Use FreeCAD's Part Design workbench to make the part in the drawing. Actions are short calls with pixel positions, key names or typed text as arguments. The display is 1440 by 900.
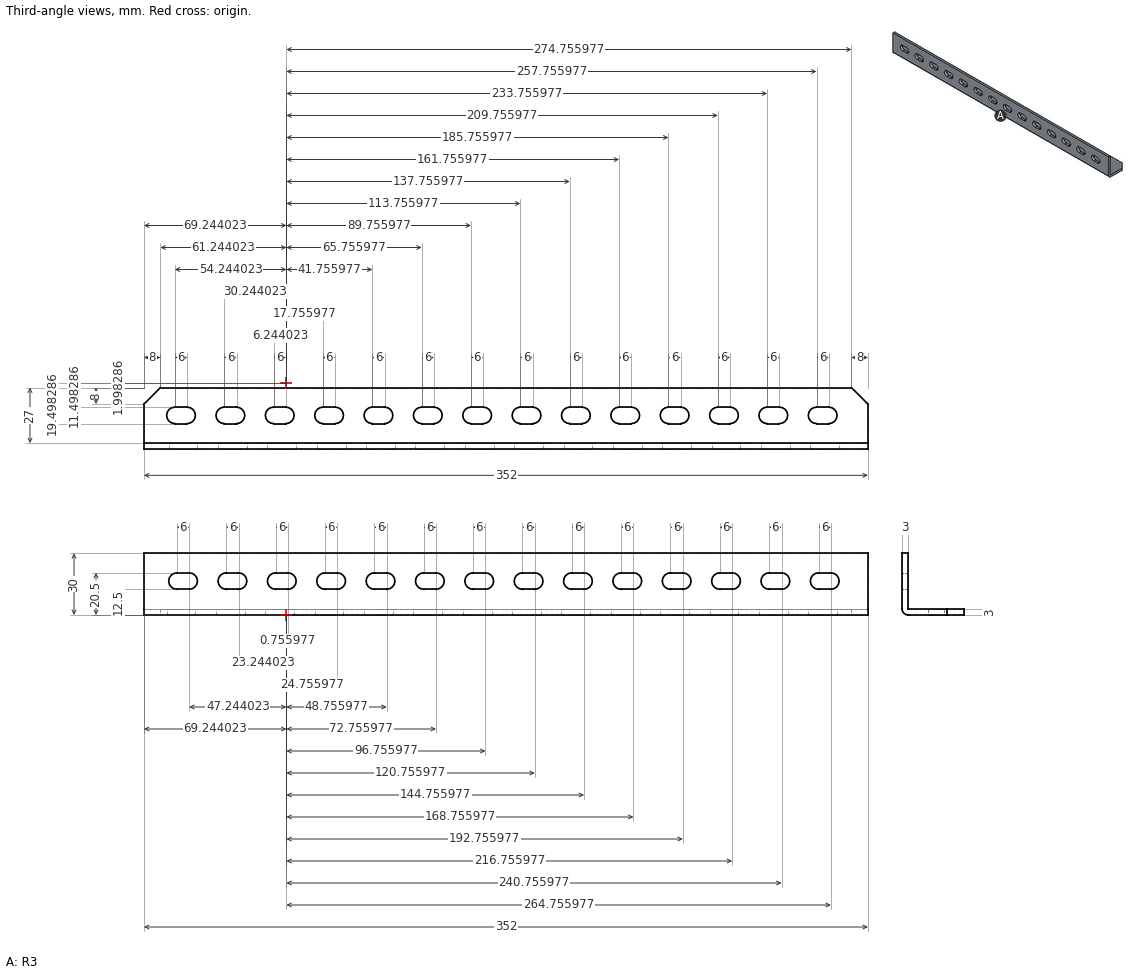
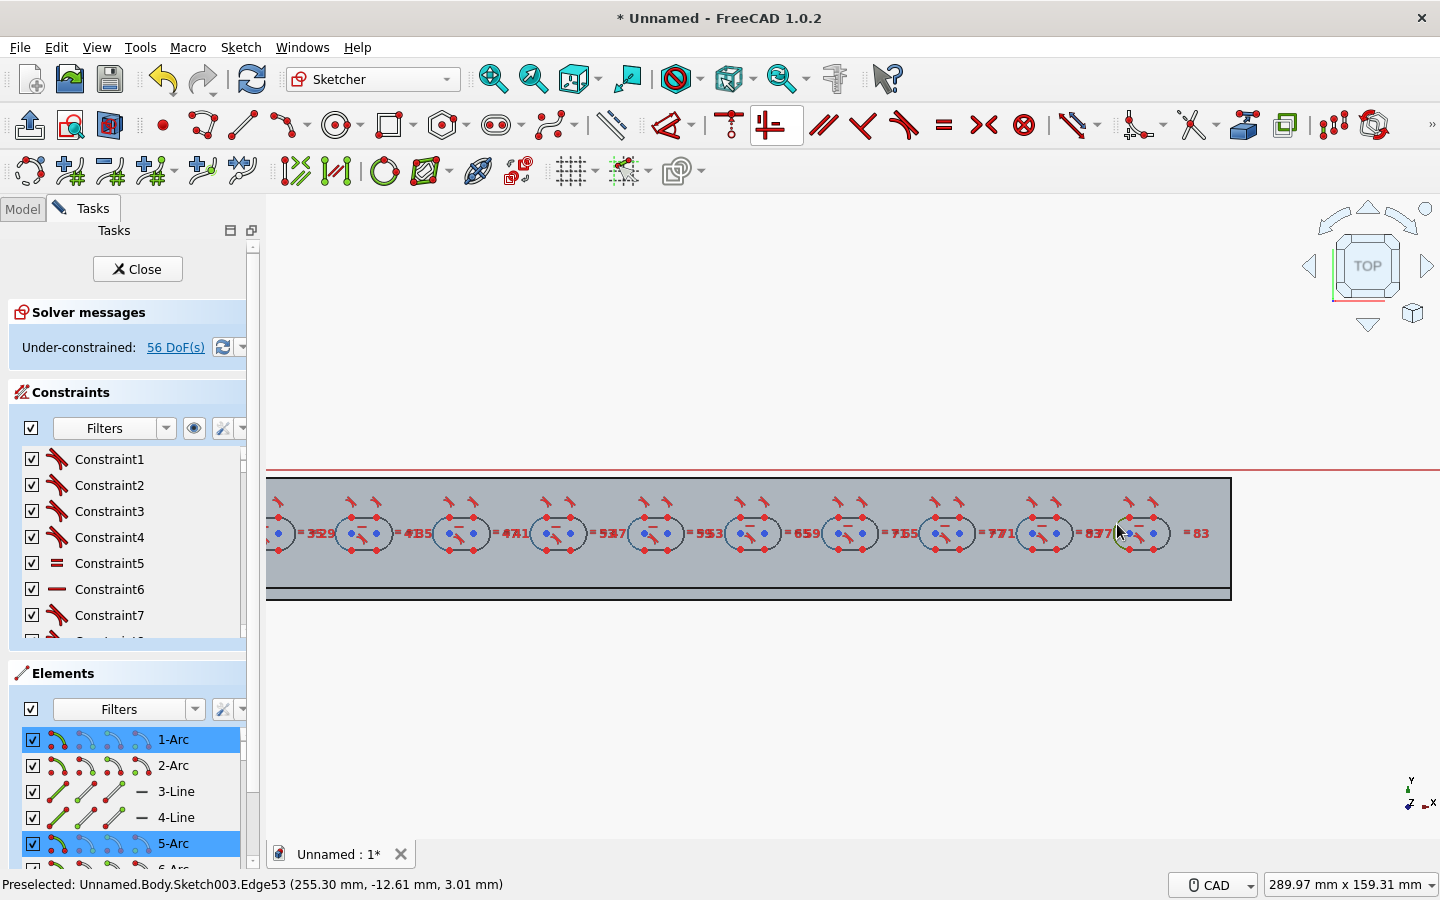
click(944, 126)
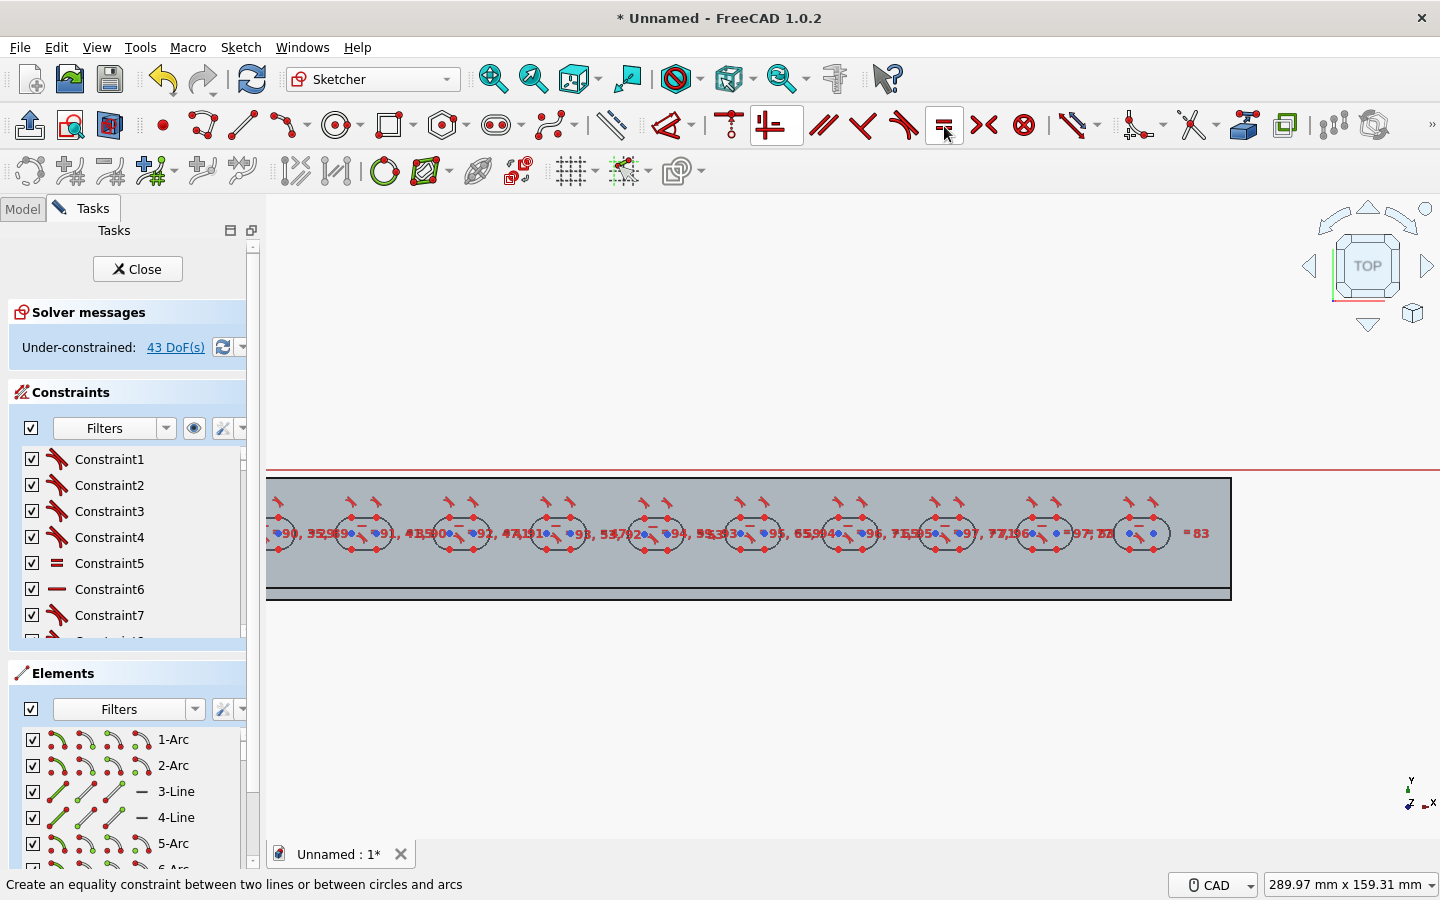
click(666, 126)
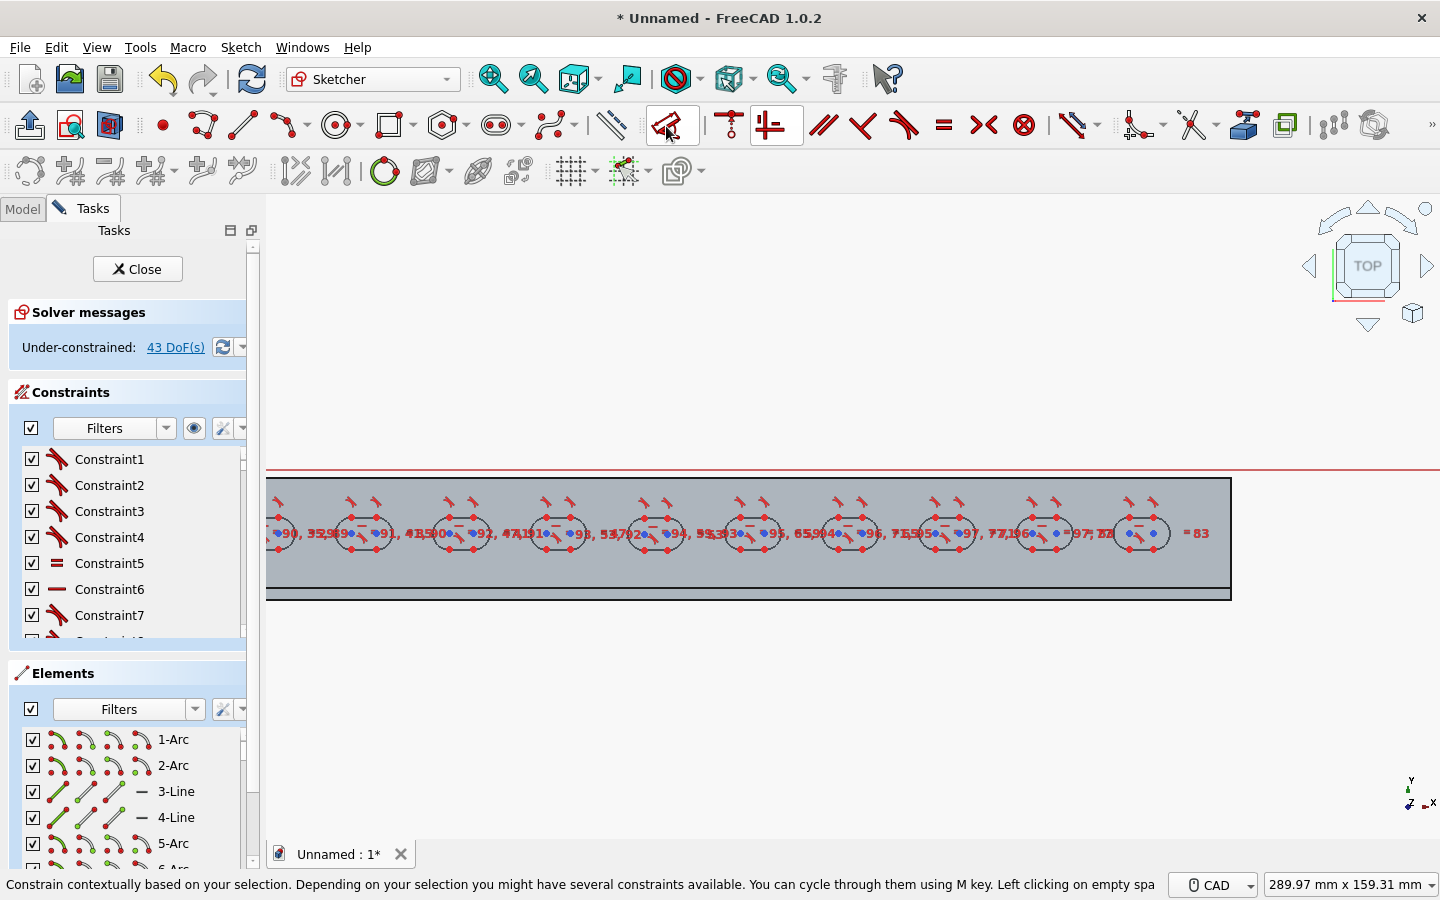
scroll(1118, 525, down, 3)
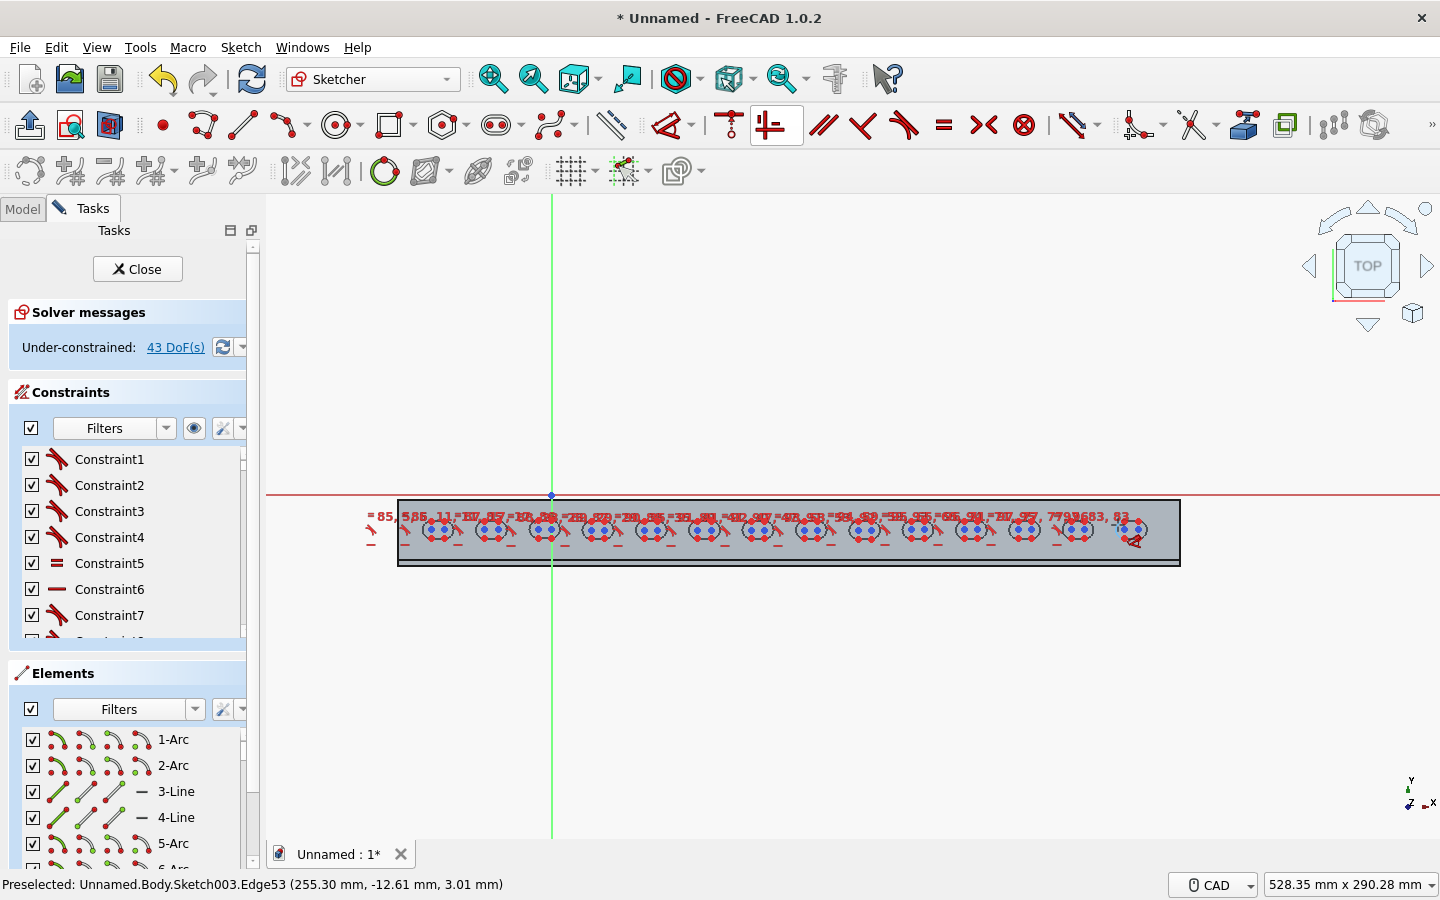
scroll(437, 521, up, 6)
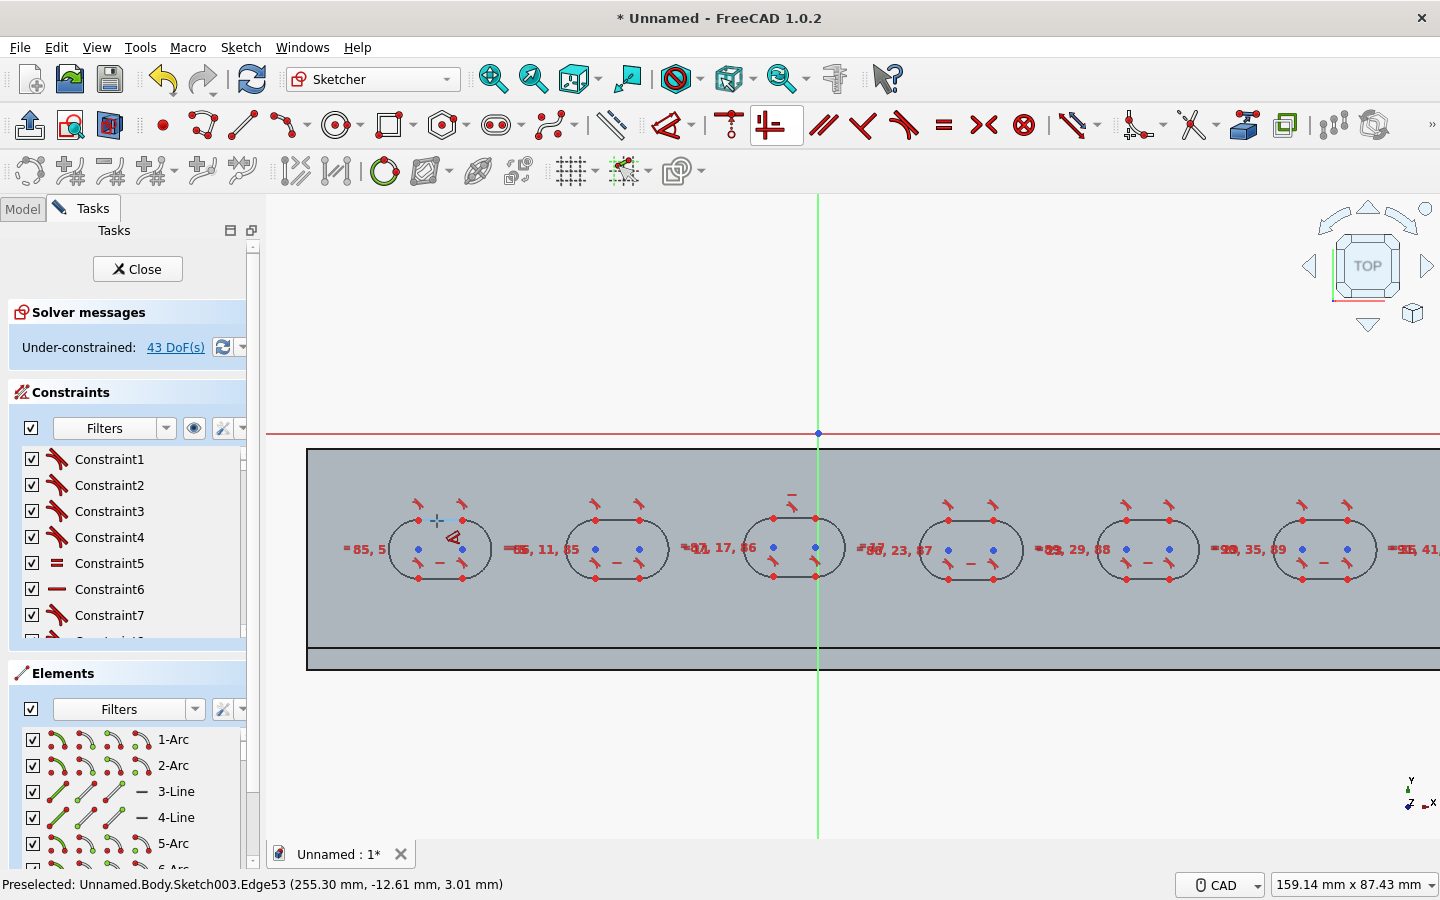
click(436, 520)
click(440, 554)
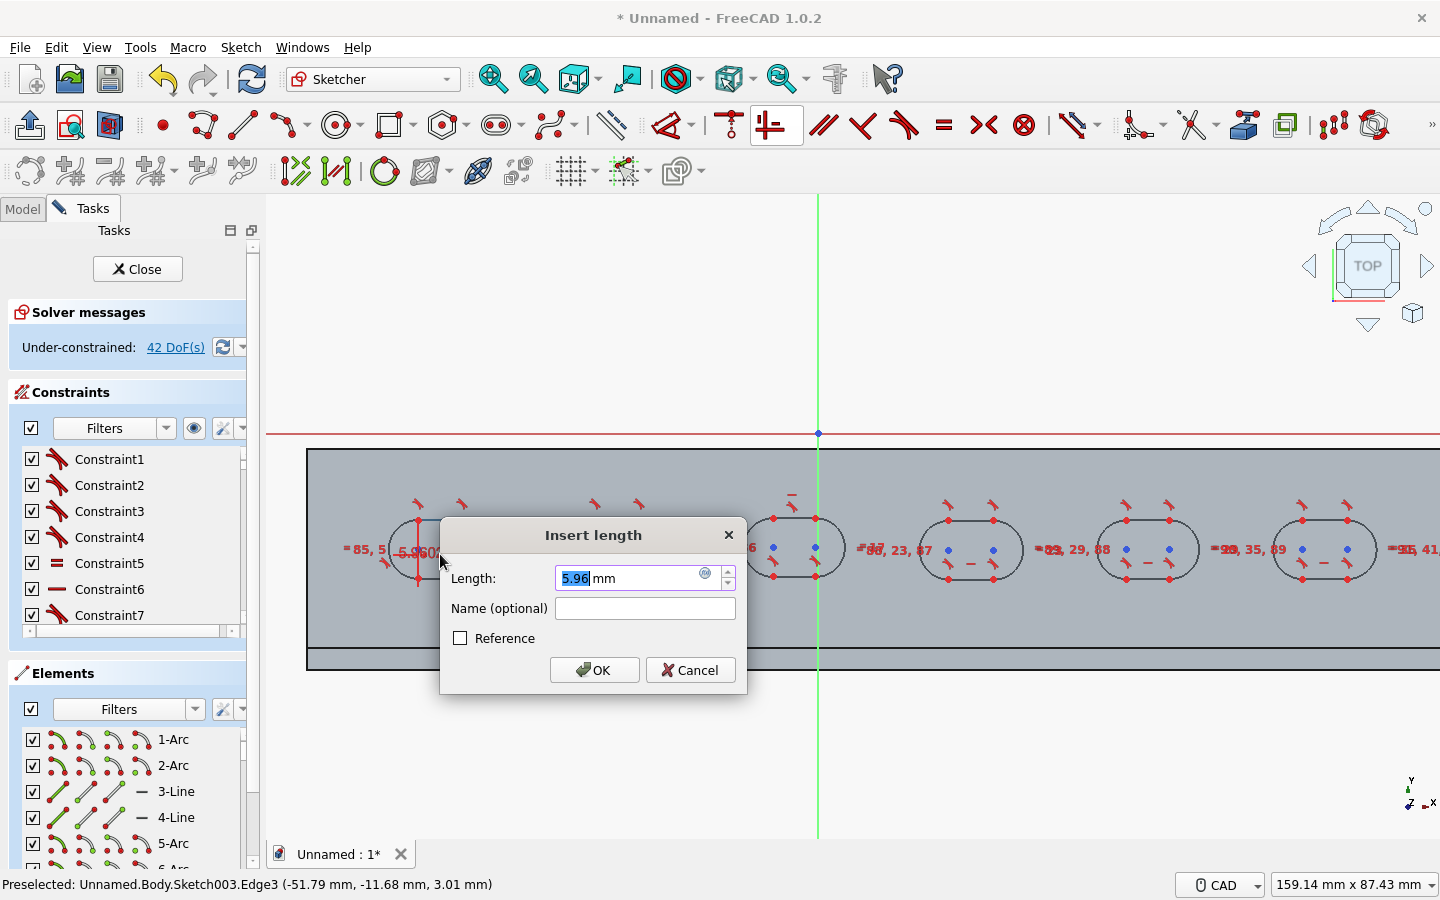
text(6)
key(Return)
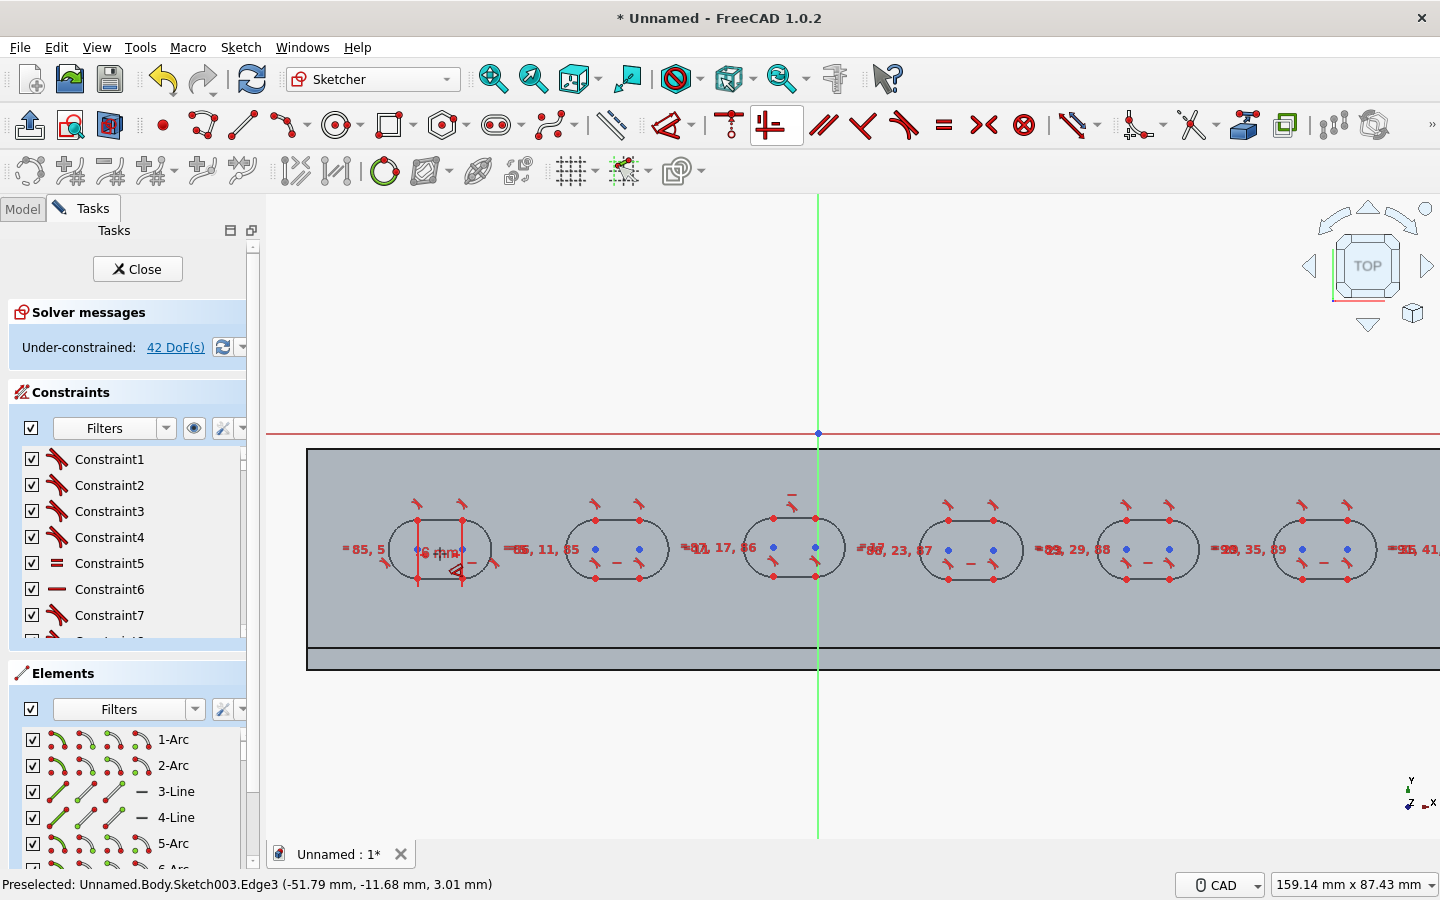
click(608, 520)
click(617, 554)